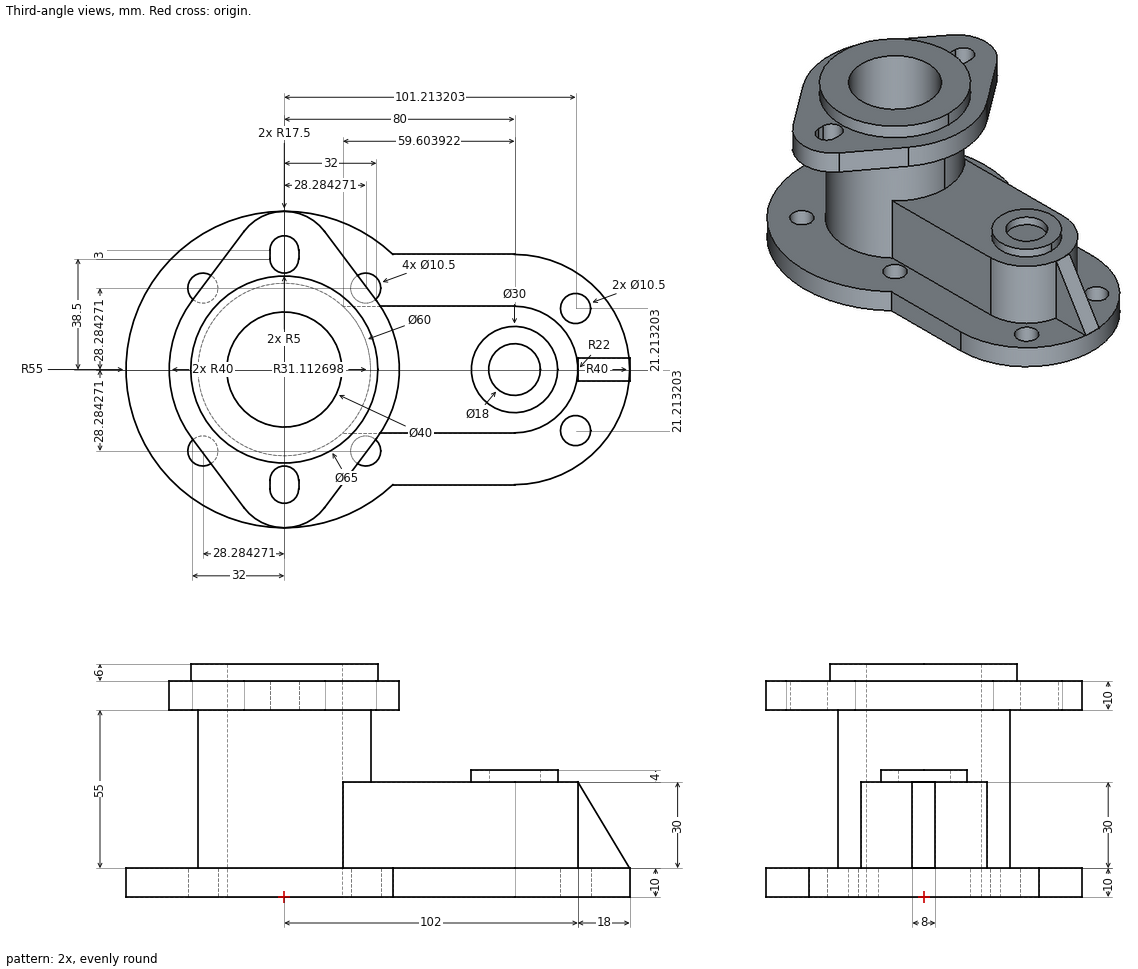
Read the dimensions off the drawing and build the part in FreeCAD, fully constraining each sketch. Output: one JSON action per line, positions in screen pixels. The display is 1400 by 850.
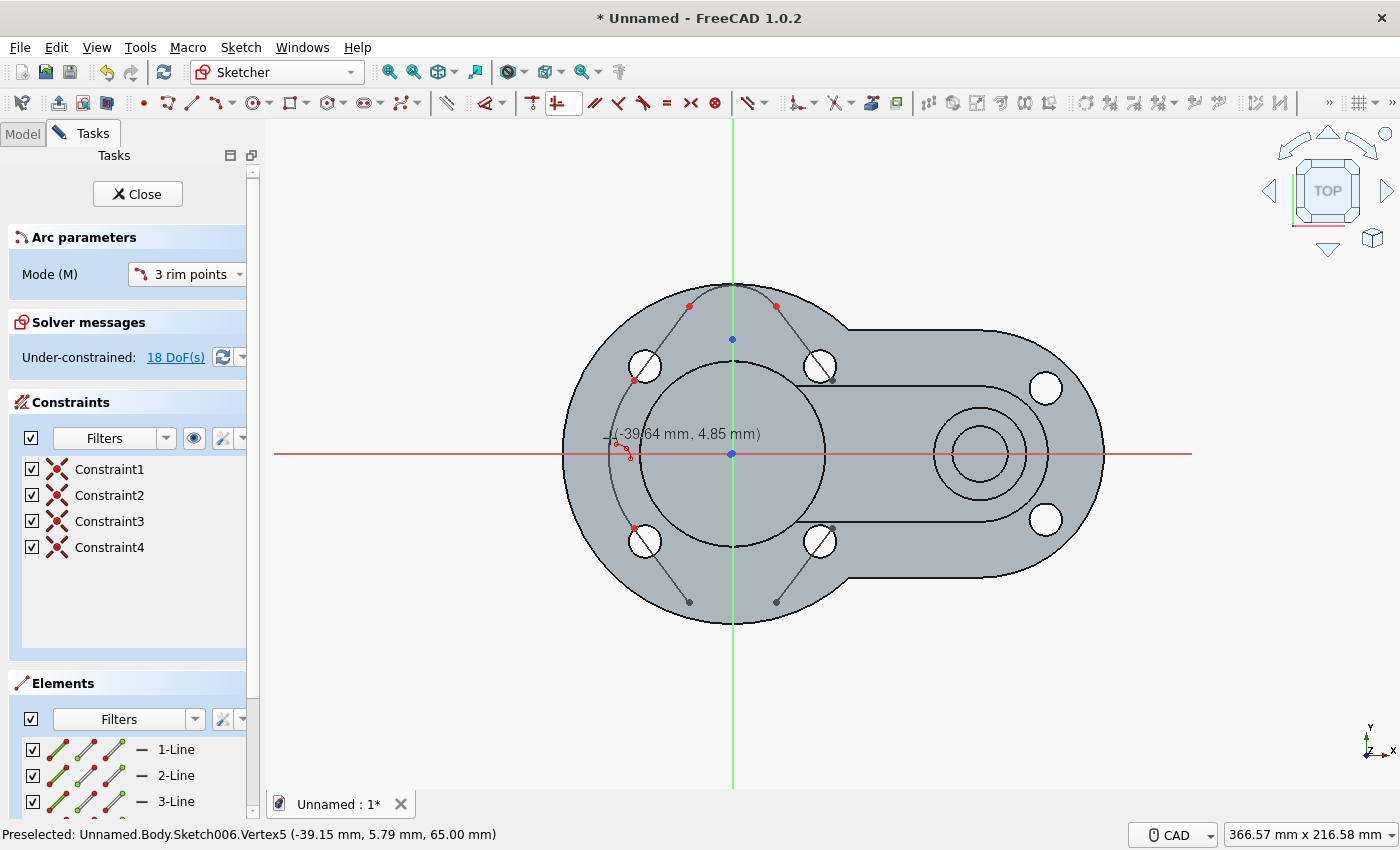
{"action": "left_click", "coordinate": [689, 603]}
{"action": "left_click", "coordinate": [776, 603]}
{"action": "left_click", "coordinate": [713, 620]}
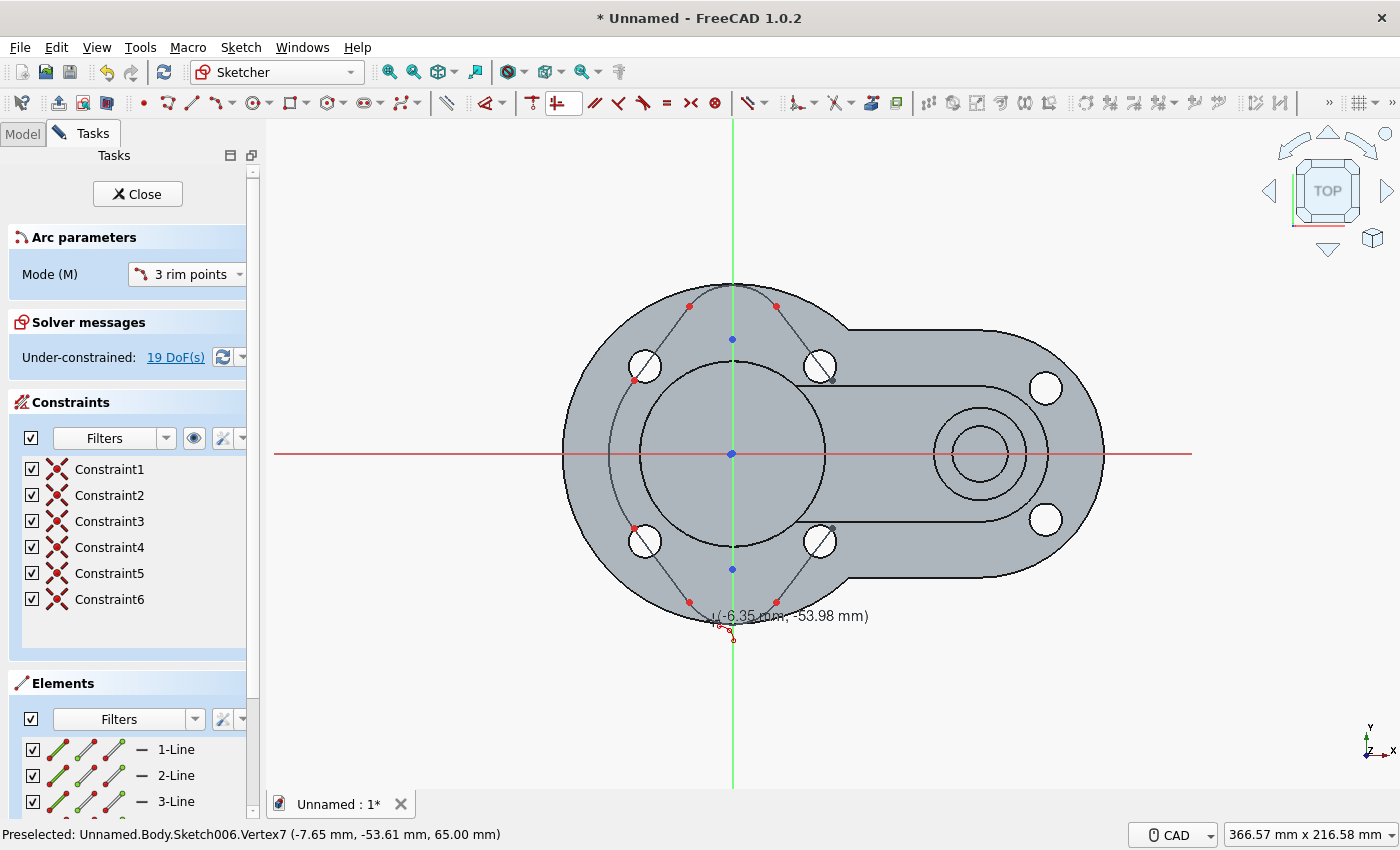
{"action": "left_click", "coordinate": [832, 529]}
{"action": "left_click", "coordinate": [832, 381]}
{"action": "left_click", "coordinate": [855, 470]}
{"action": "key", "text": "Escape"}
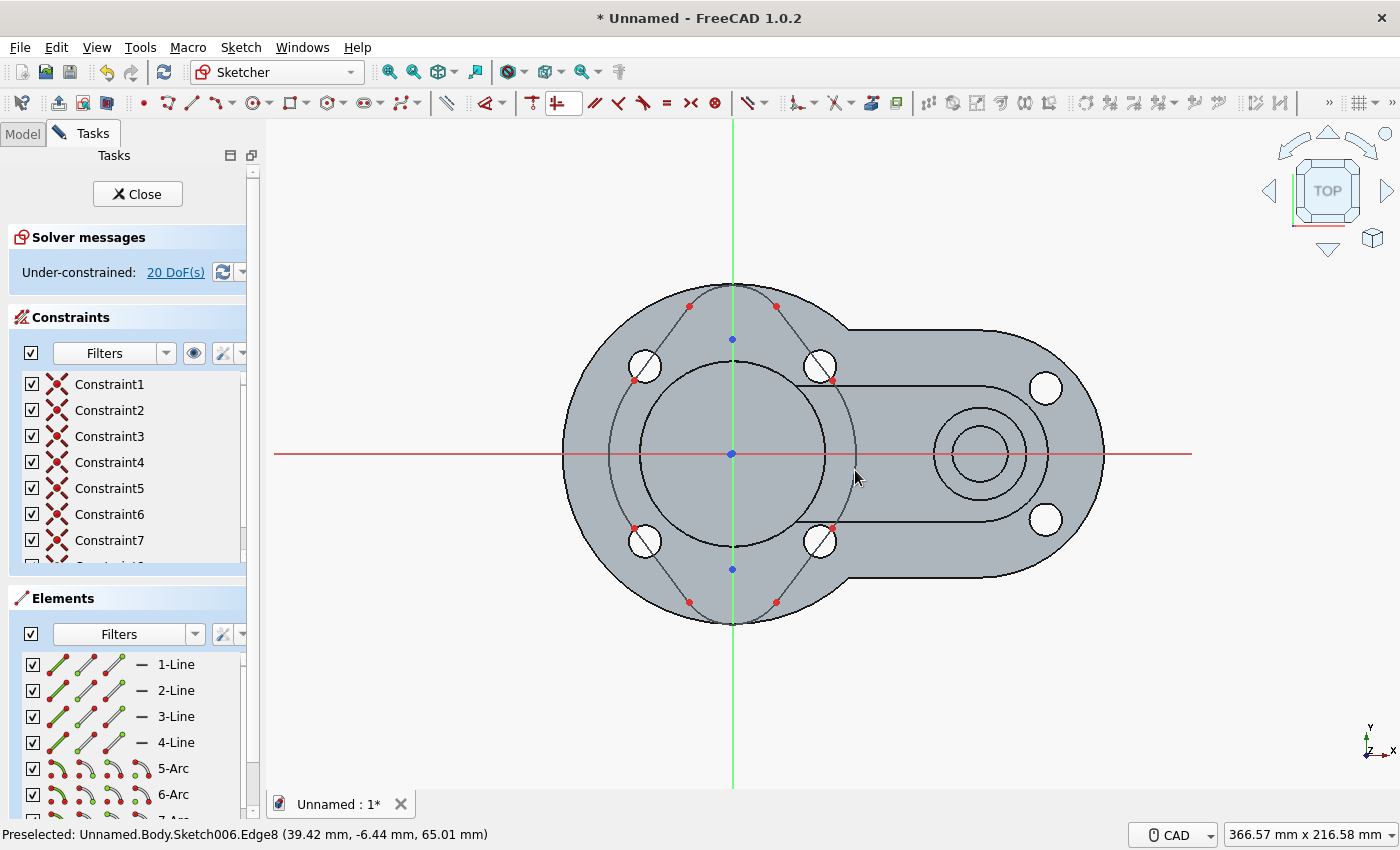
{"action": "left_click", "coordinate": [815, 359]}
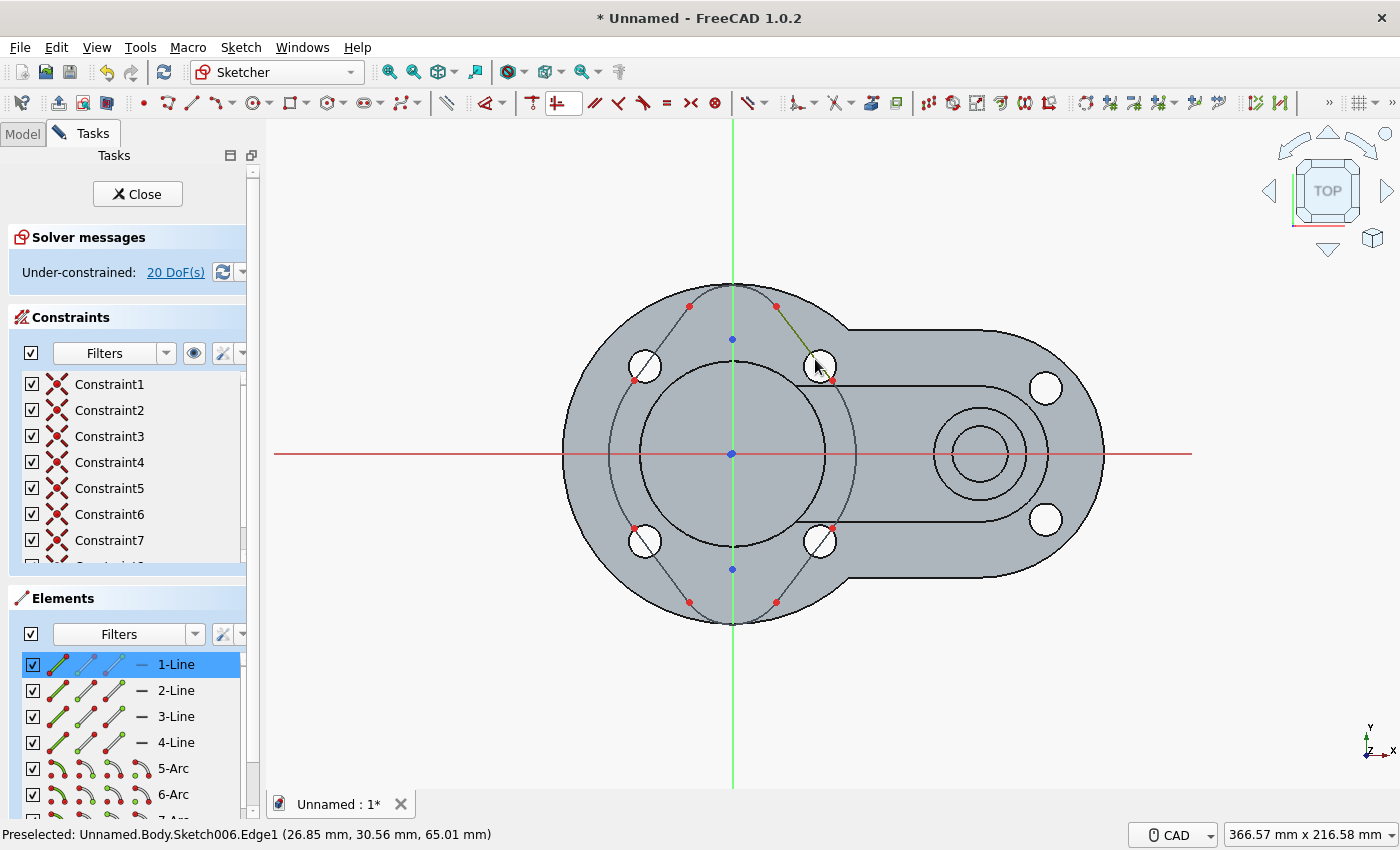
{"action": "left_click", "coordinate": [752, 289]}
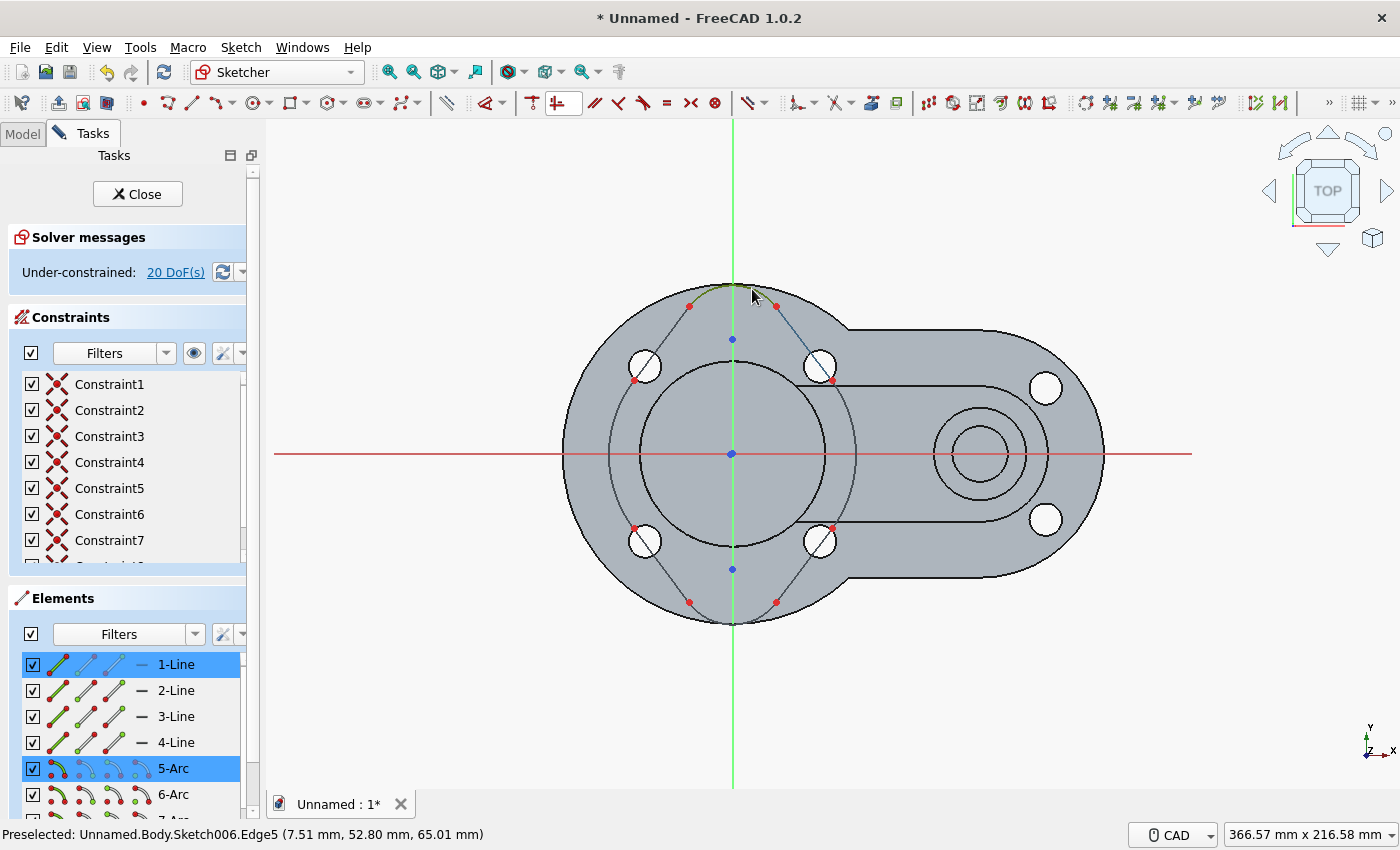
{"action": "left_click", "coordinate": [644, 104]}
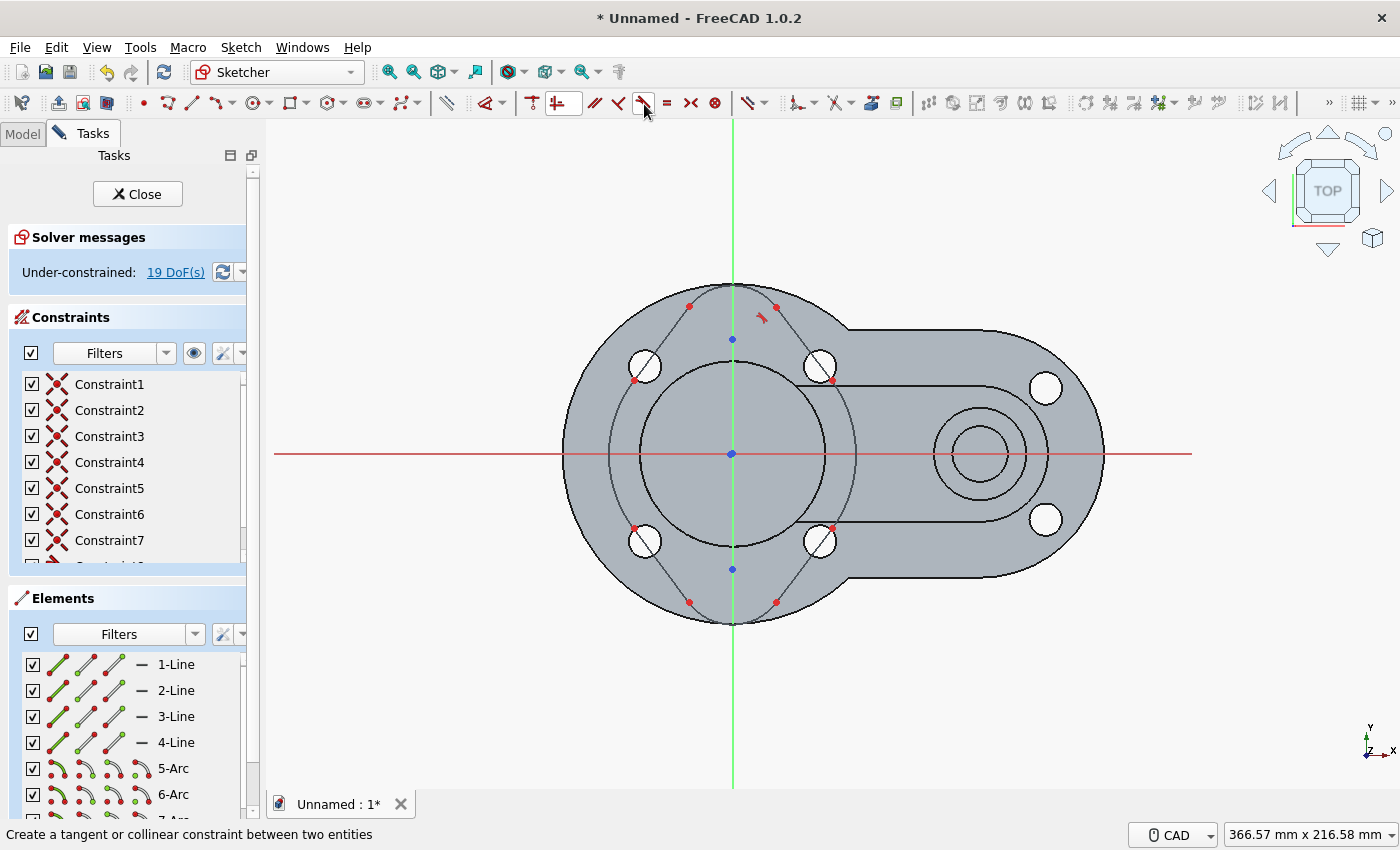
{"action": "left_click", "coordinate": [815, 359]}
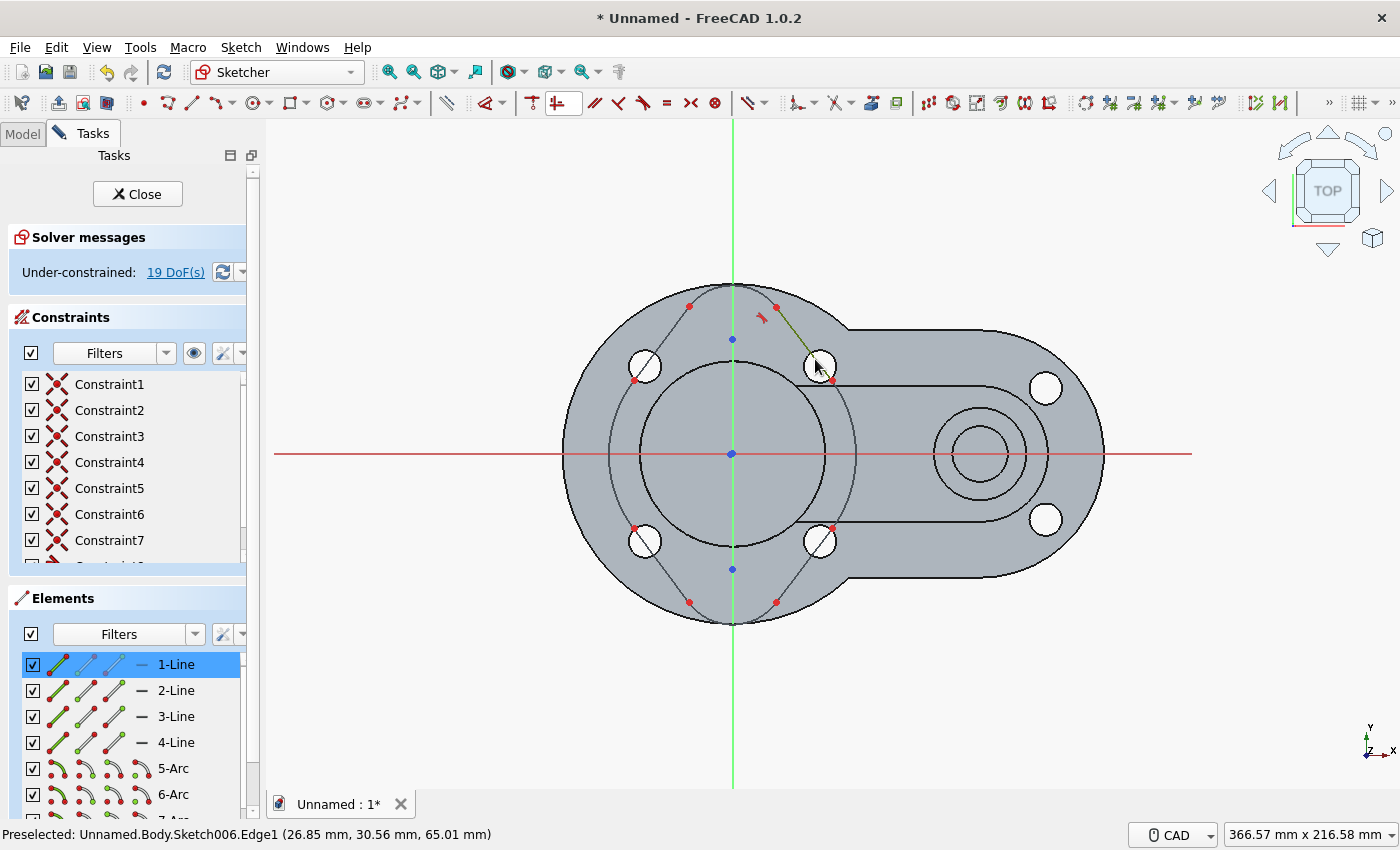
{"action": "left_click", "coordinate": [852, 486]}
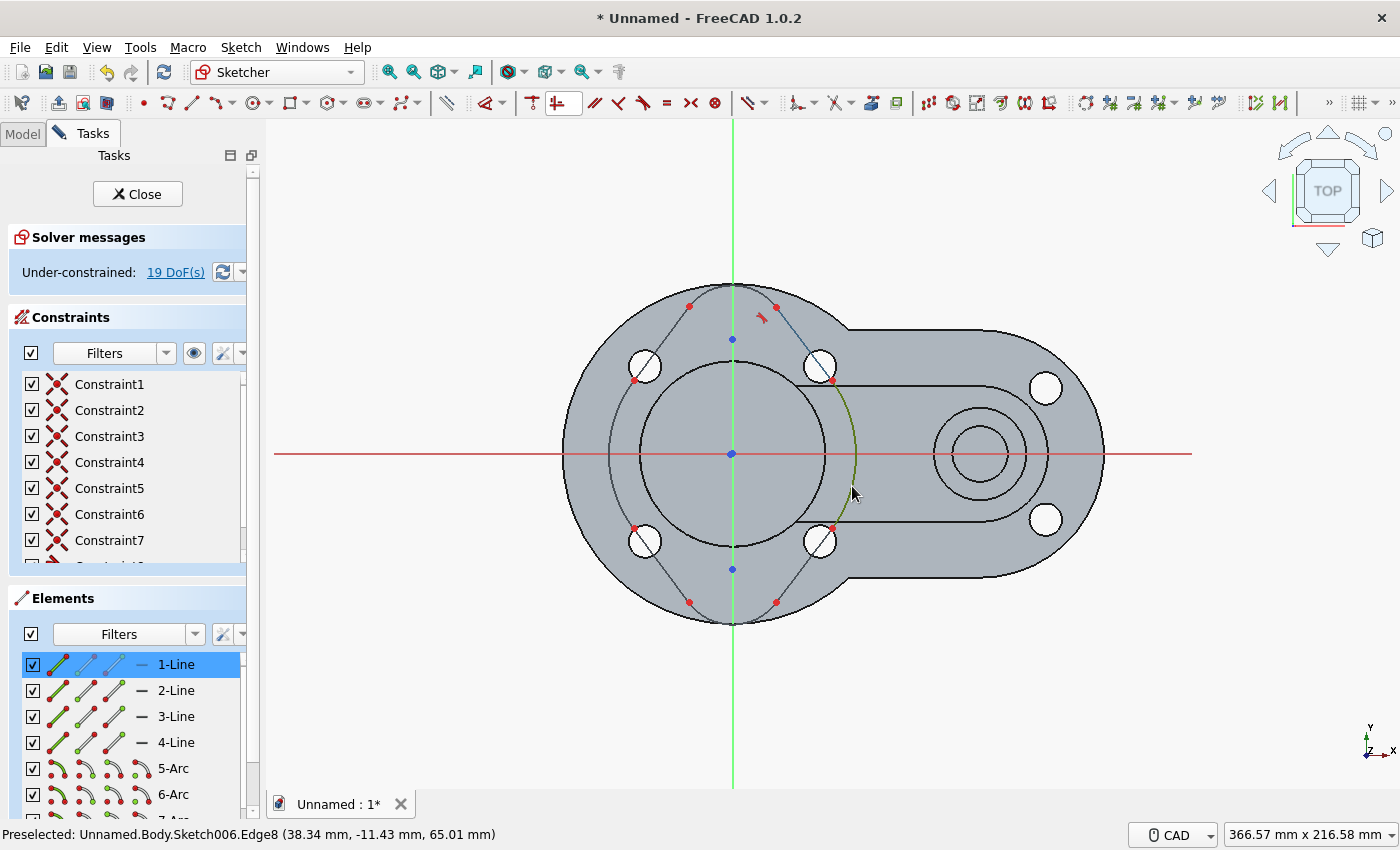
{"action": "left_click", "coordinate": [644, 104]}